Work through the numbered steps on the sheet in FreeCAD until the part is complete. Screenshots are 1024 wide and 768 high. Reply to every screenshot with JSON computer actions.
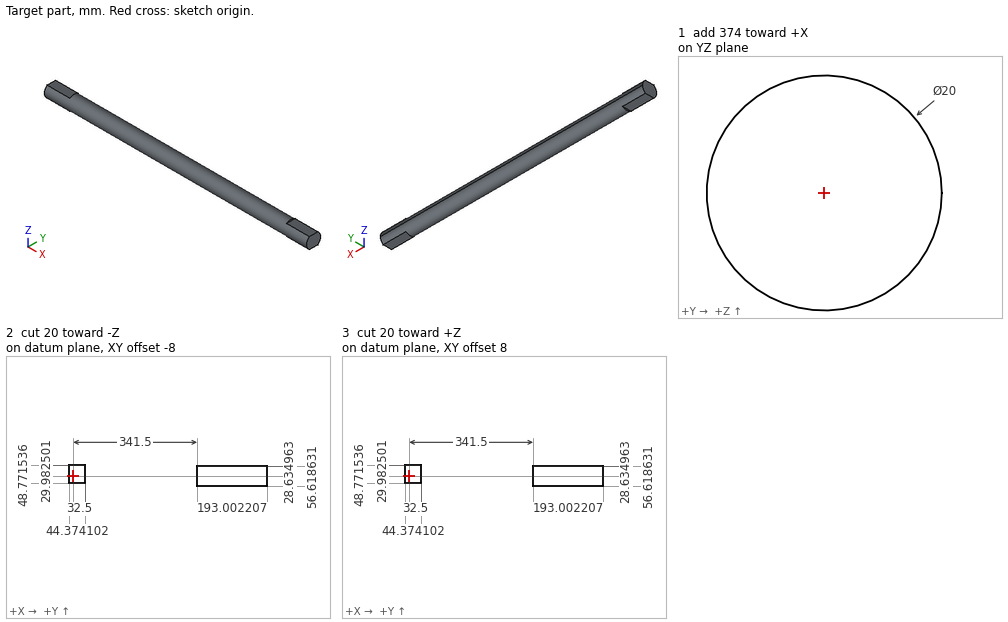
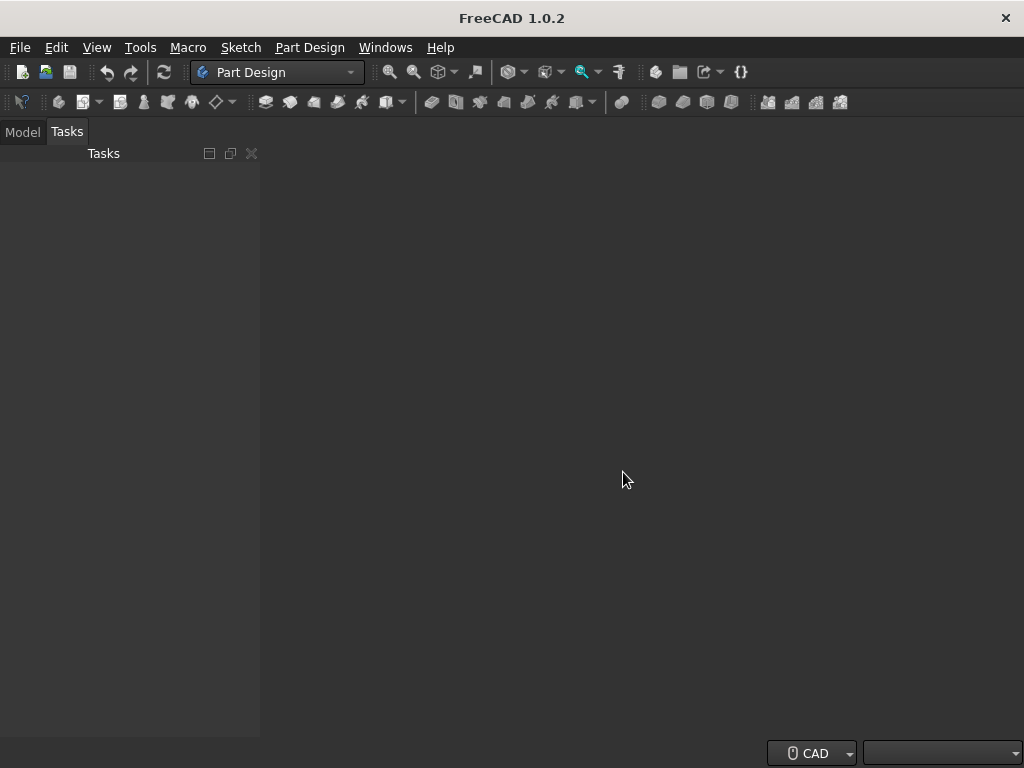
{"action": "left_click", "coordinate": [22, 72]}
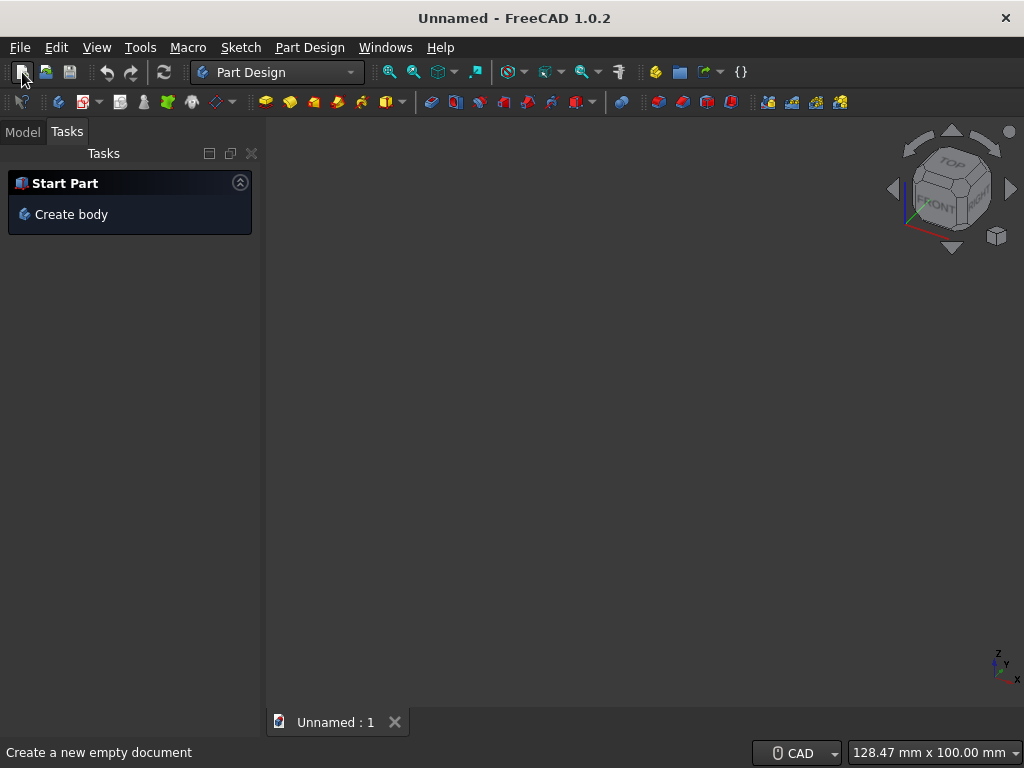
{"action": "left_click", "coordinate": [84, 102]}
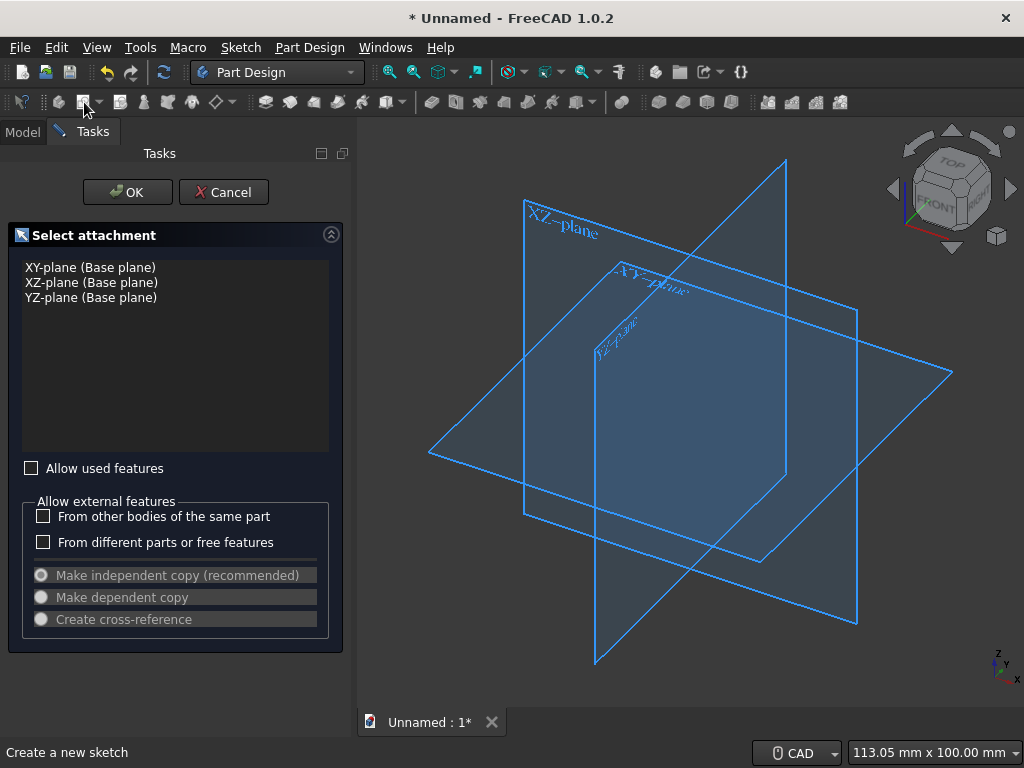
{"action": "left_click", "coordinate": [82, 298]}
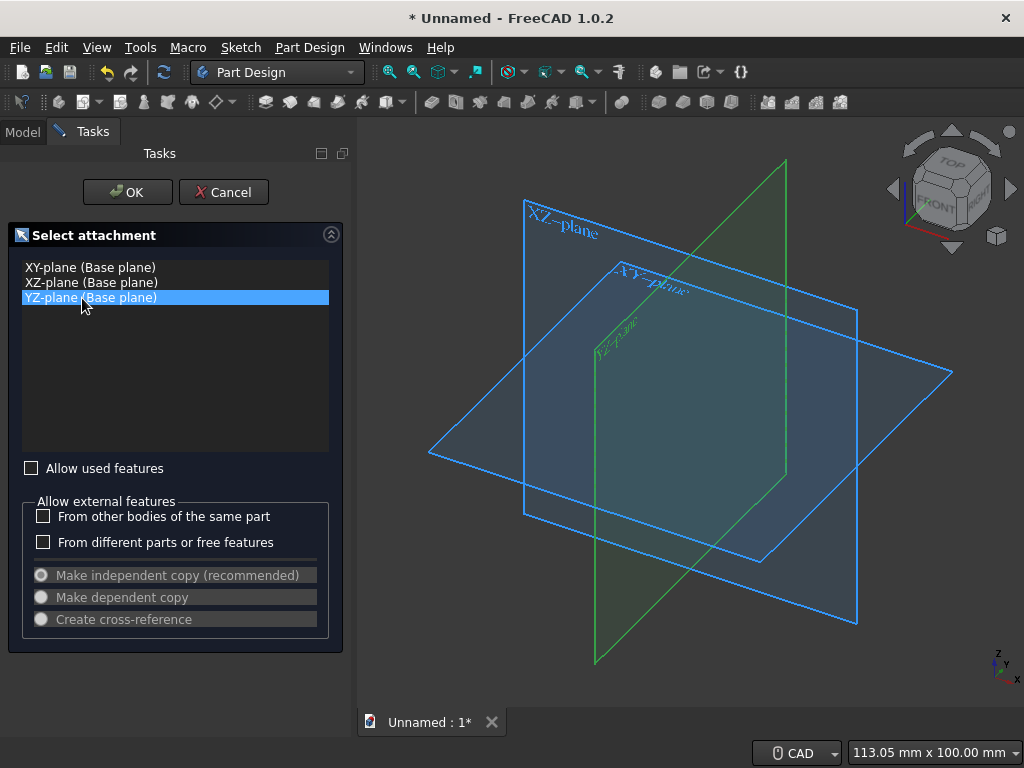
{"action": "left_click", "coordinate": [128, 192]}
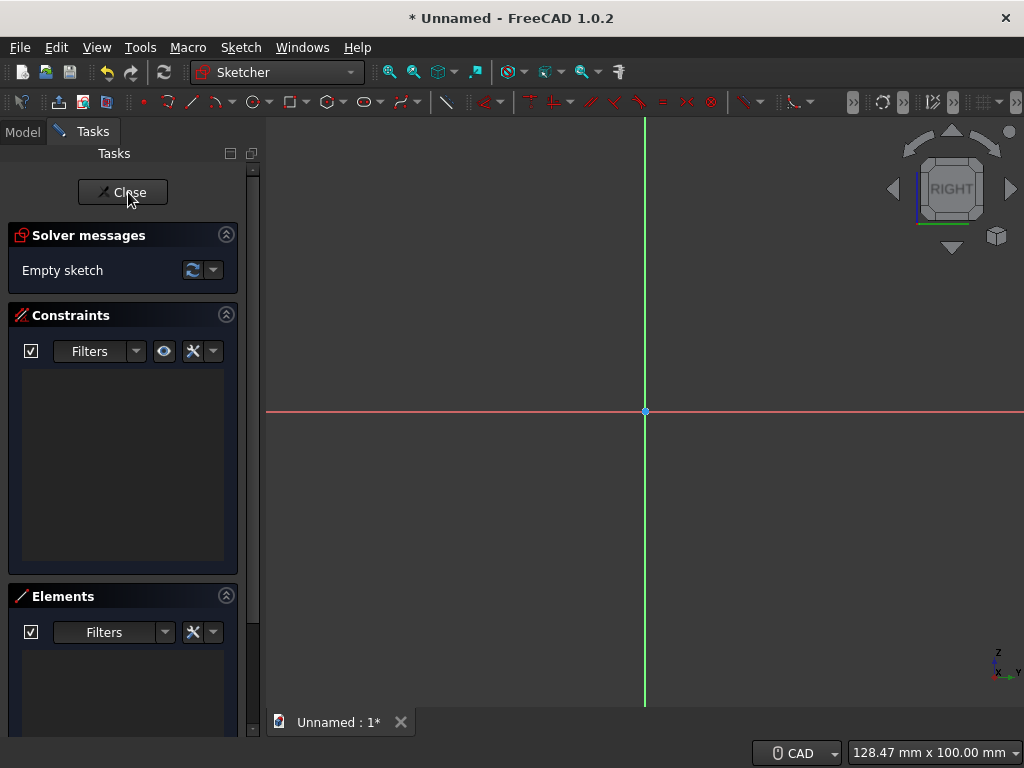
{"action": "scroll", "coordinate": [675, 412], "scroll_direction": "up", "scroll_amount": 6}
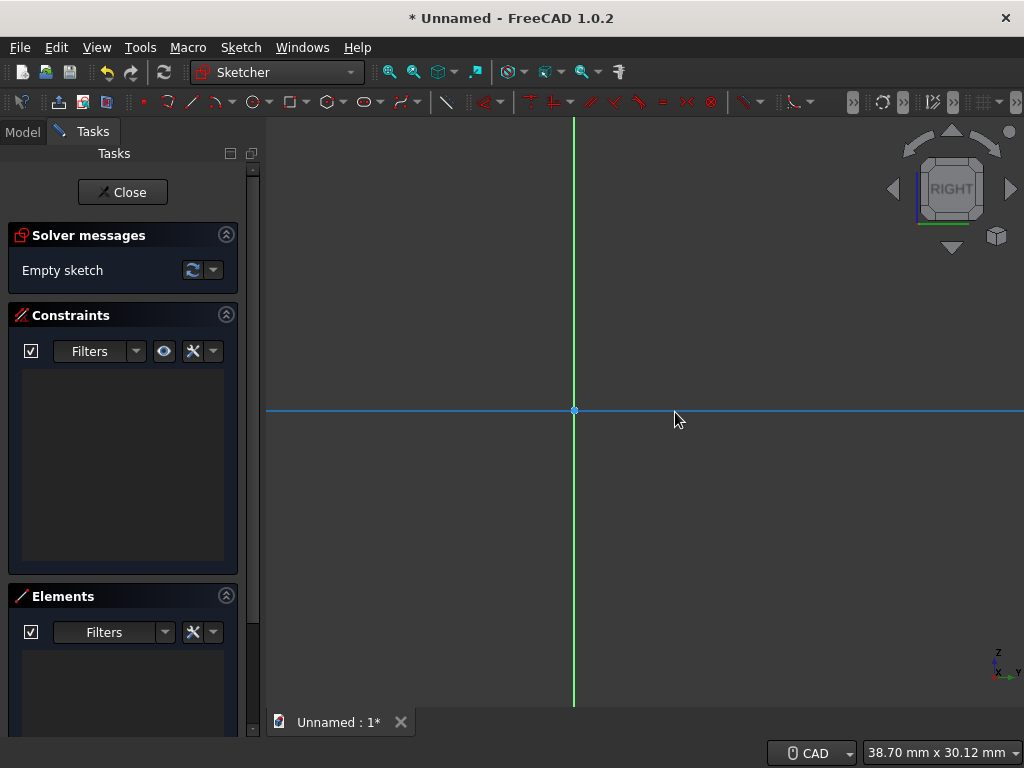
{"action": "key", "text": "g c"}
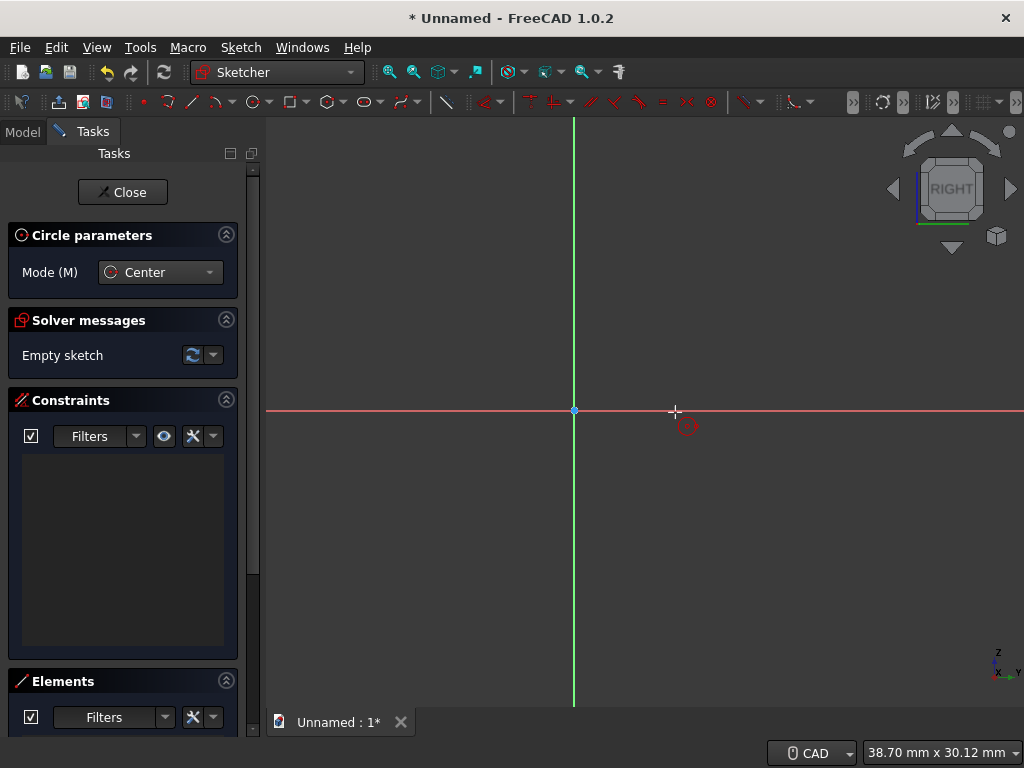
{"action": "left_click", "coordinate": [574, 411]}
{"action": "mouse_move", "coordinate": [713, 272]}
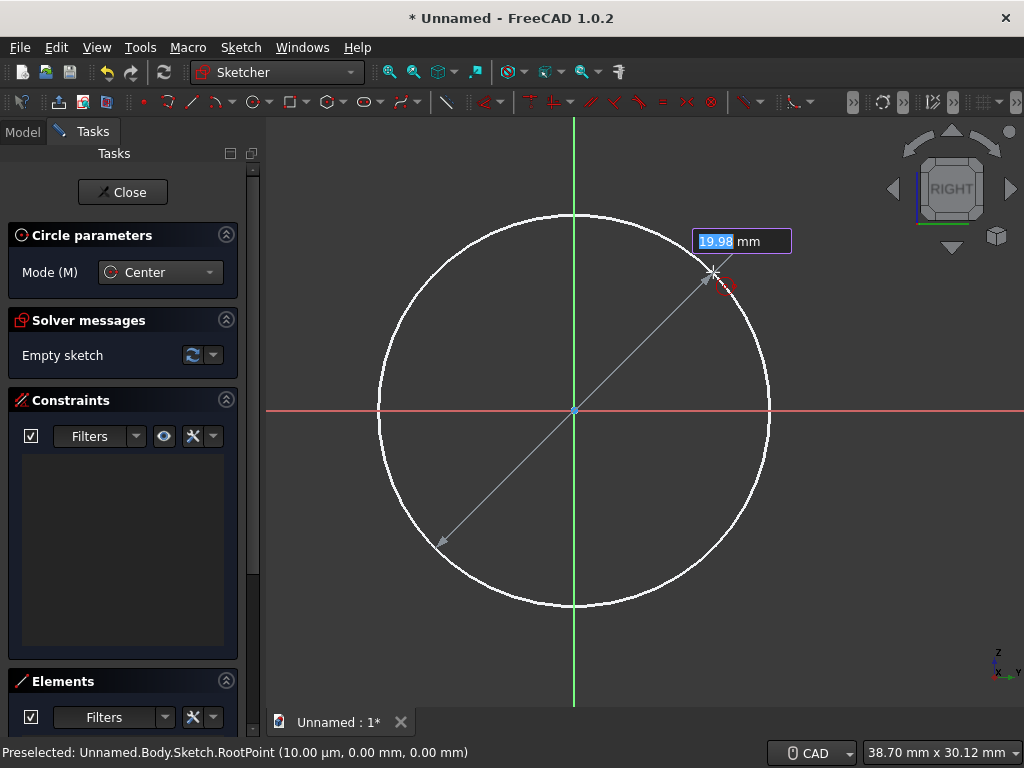
{"action": "type", "text": "20"}
{"action": "key", "text": "Return"}
{"action": "key", "text": "Escape"}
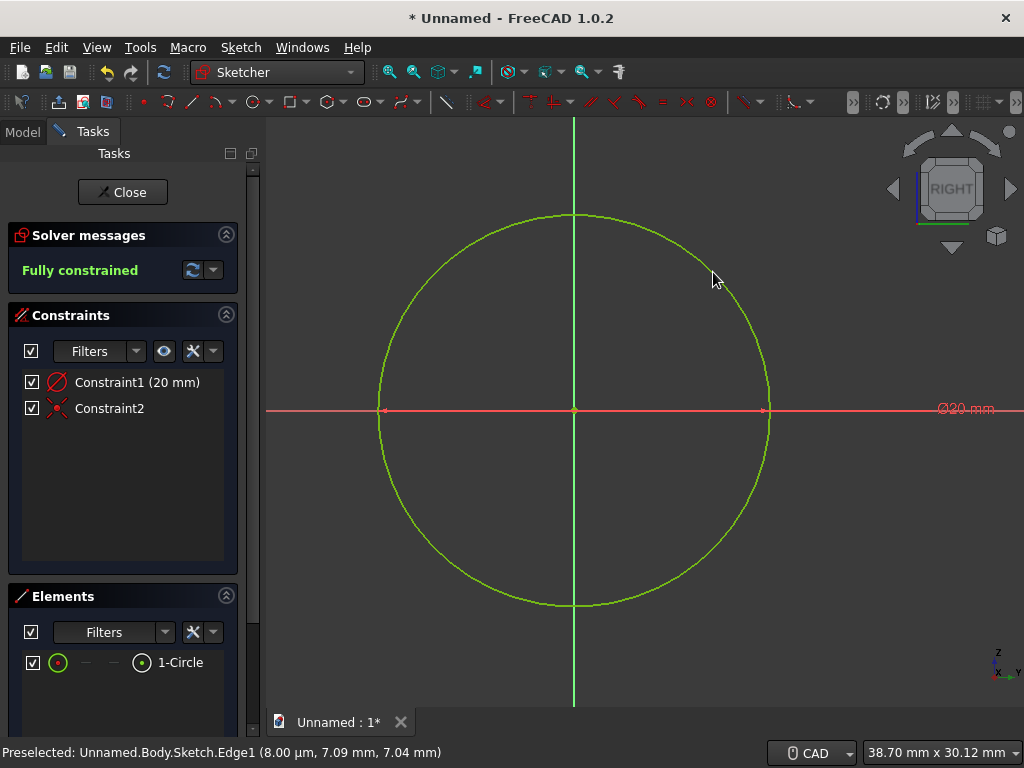
{"action": "left_click", "coordinate": [123, 192]}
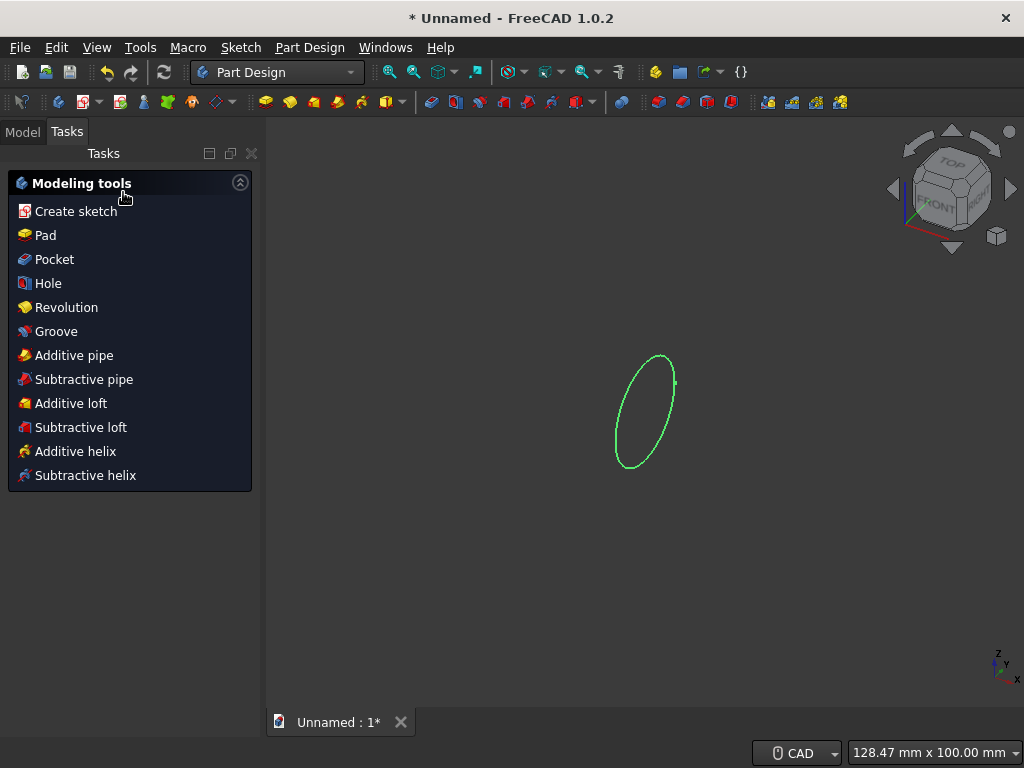
{"action": "left_click", "coordinate": [266, 102]}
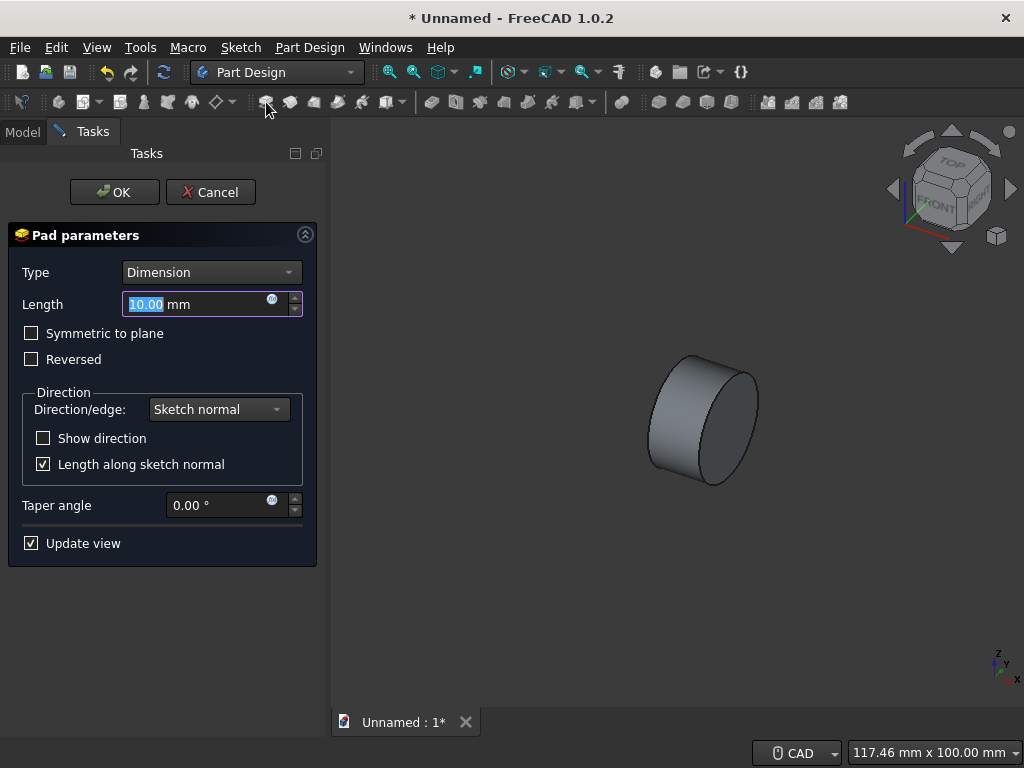
{"action": "type", "text": "374"}
{"action": "key", "text": "Tab"}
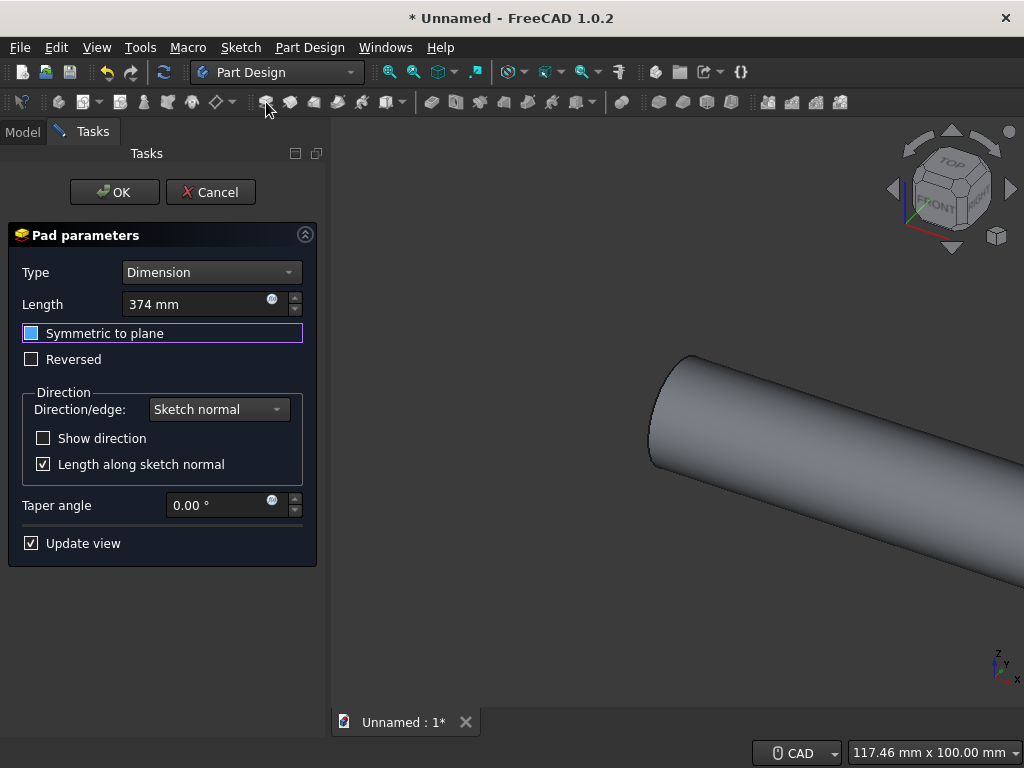
{"action": "left_click", "coordinate": [115, 192]}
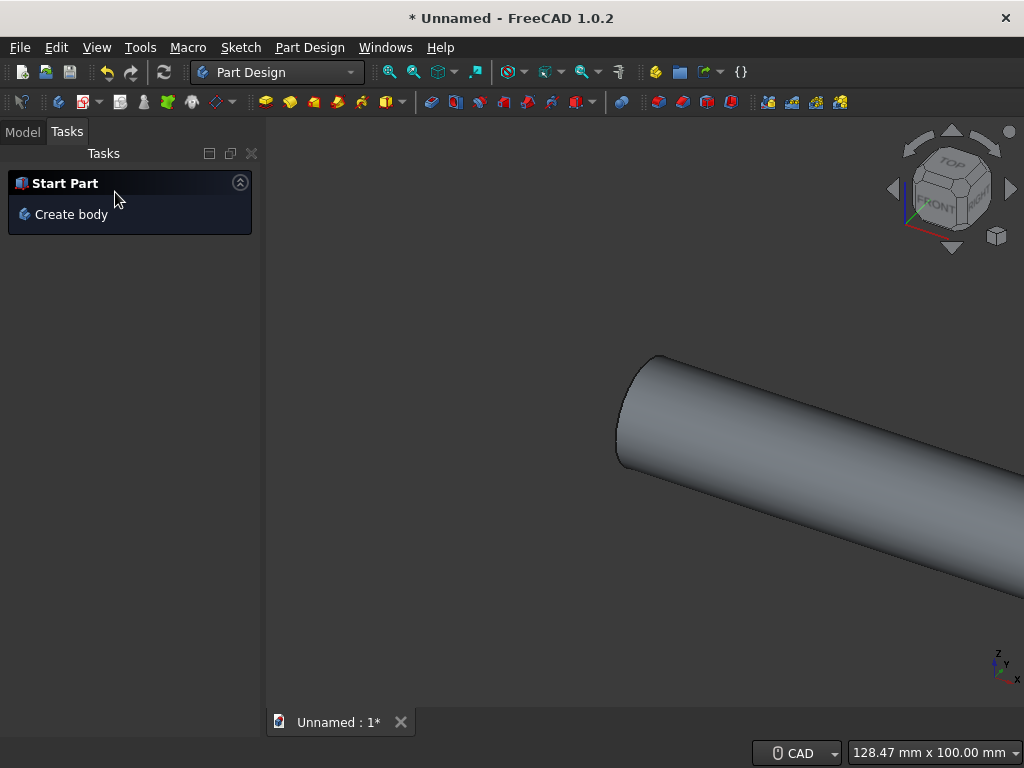
{"action": "left_click", "coordinate": [390, 72]}